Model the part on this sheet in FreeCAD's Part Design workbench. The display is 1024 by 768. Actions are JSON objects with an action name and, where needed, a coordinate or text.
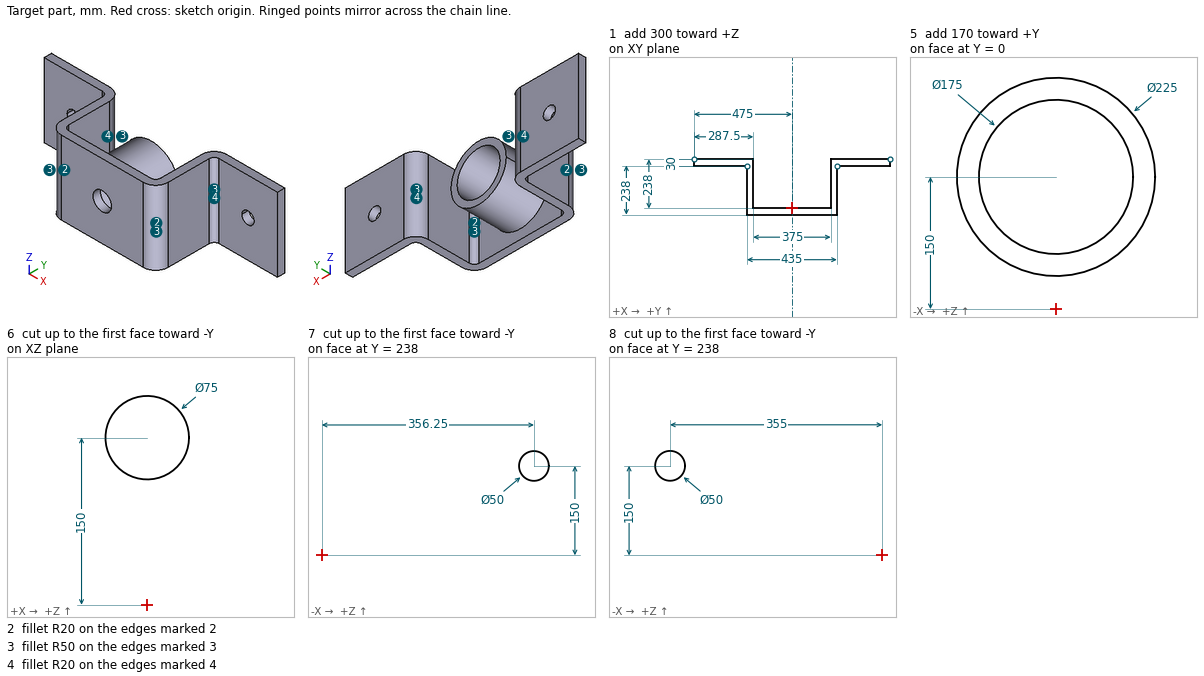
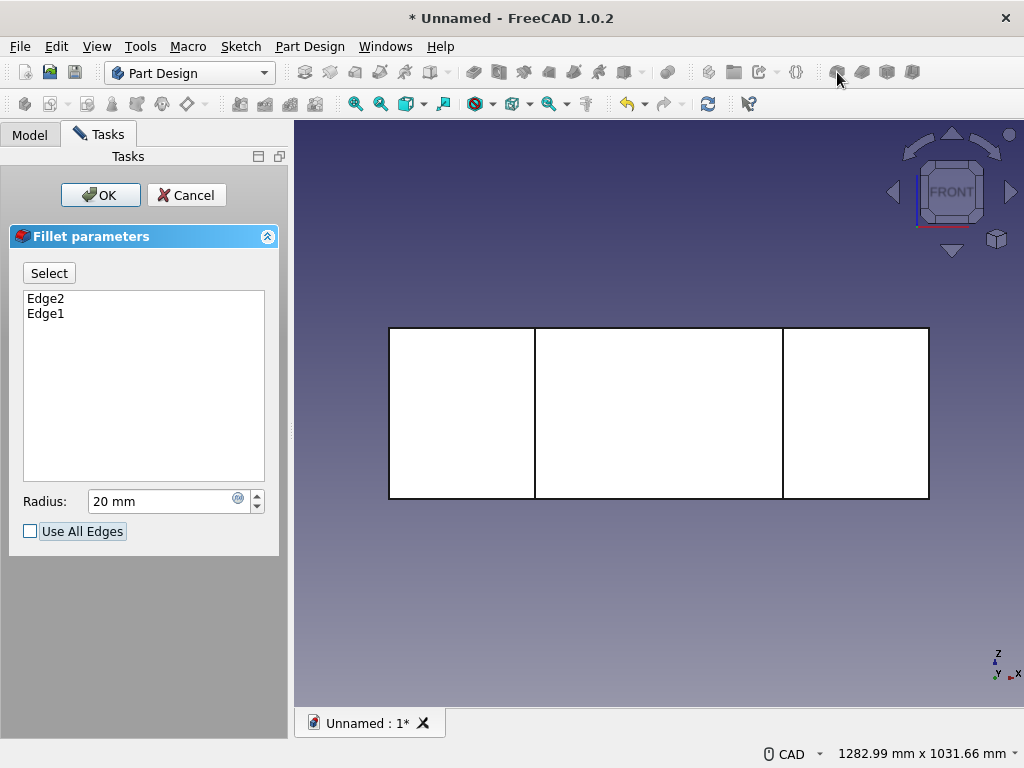
{"action": "left_click", "coordinate": [101, 195]}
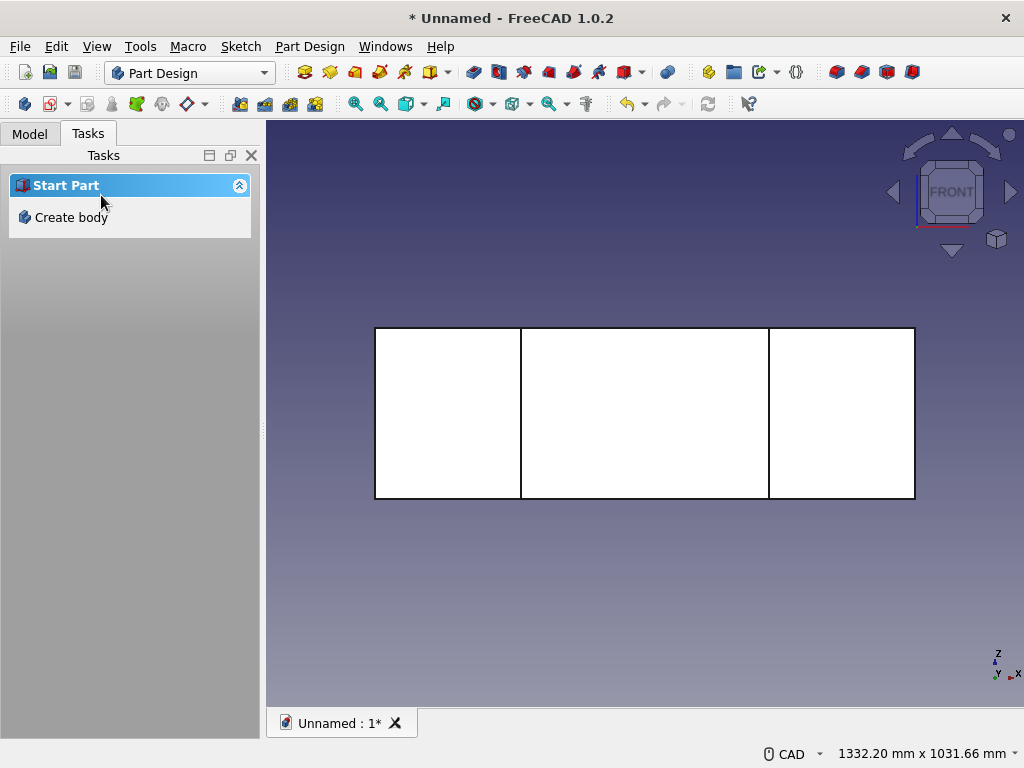
{"action": "left_click", "coordinate": [769, 412]}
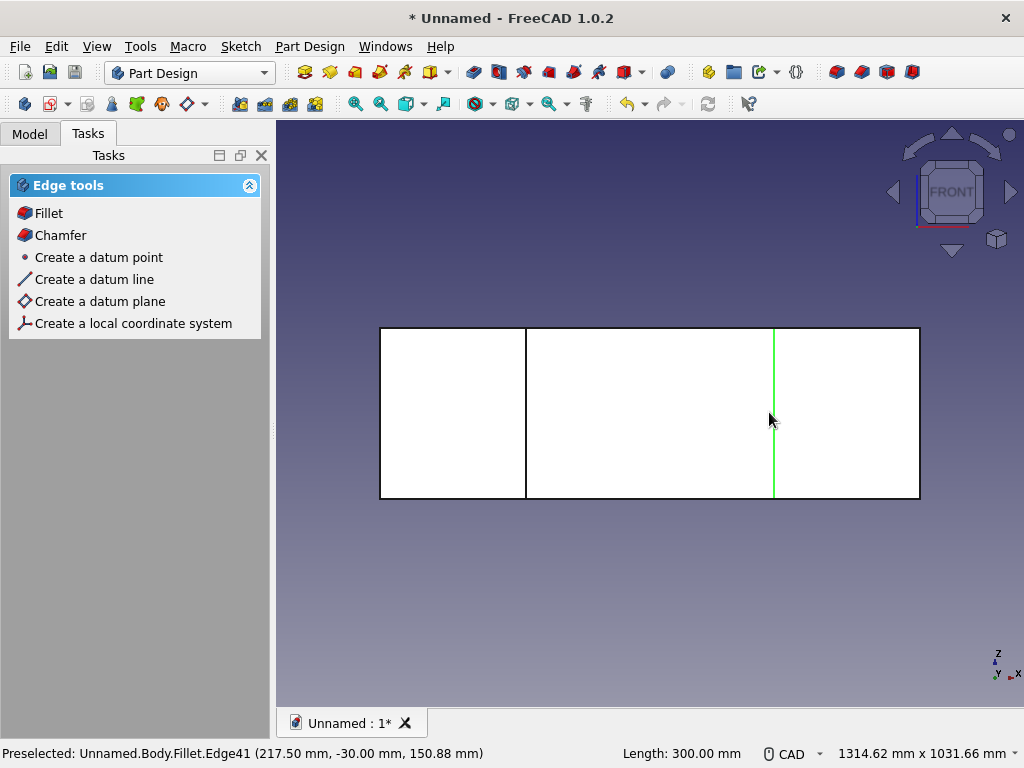
{"action": "left_click", "coordinate": [526, 412], "text": "ctrl"}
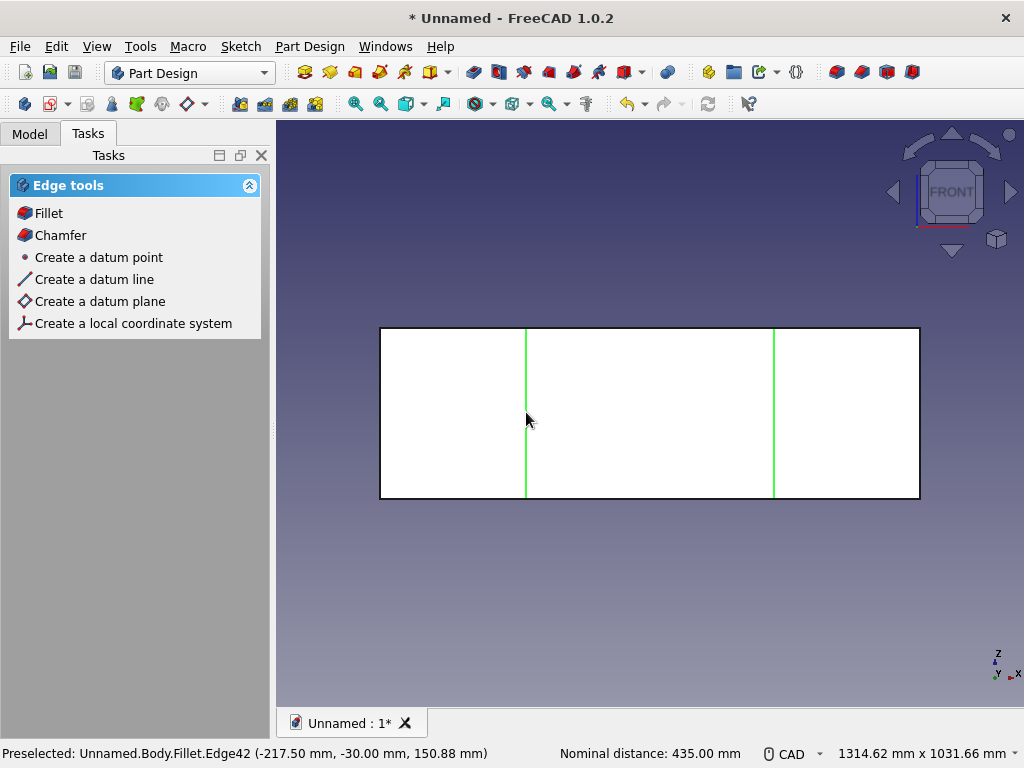
{"action": "key", "text": "0"}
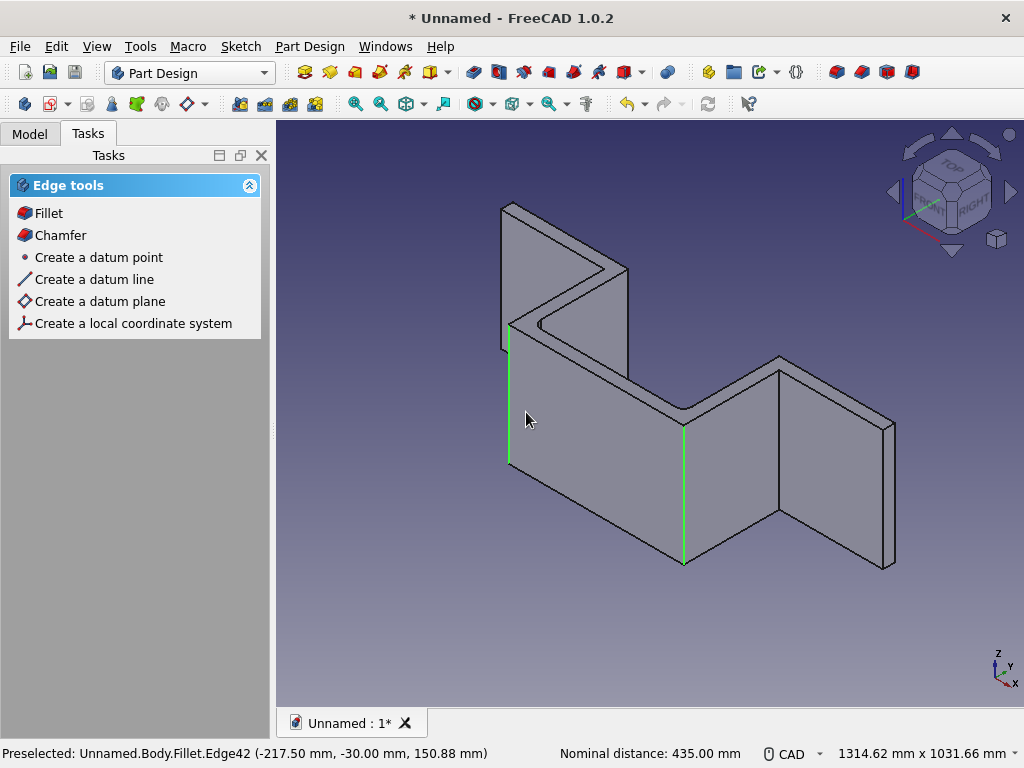
{"action": "key", "text": "2"}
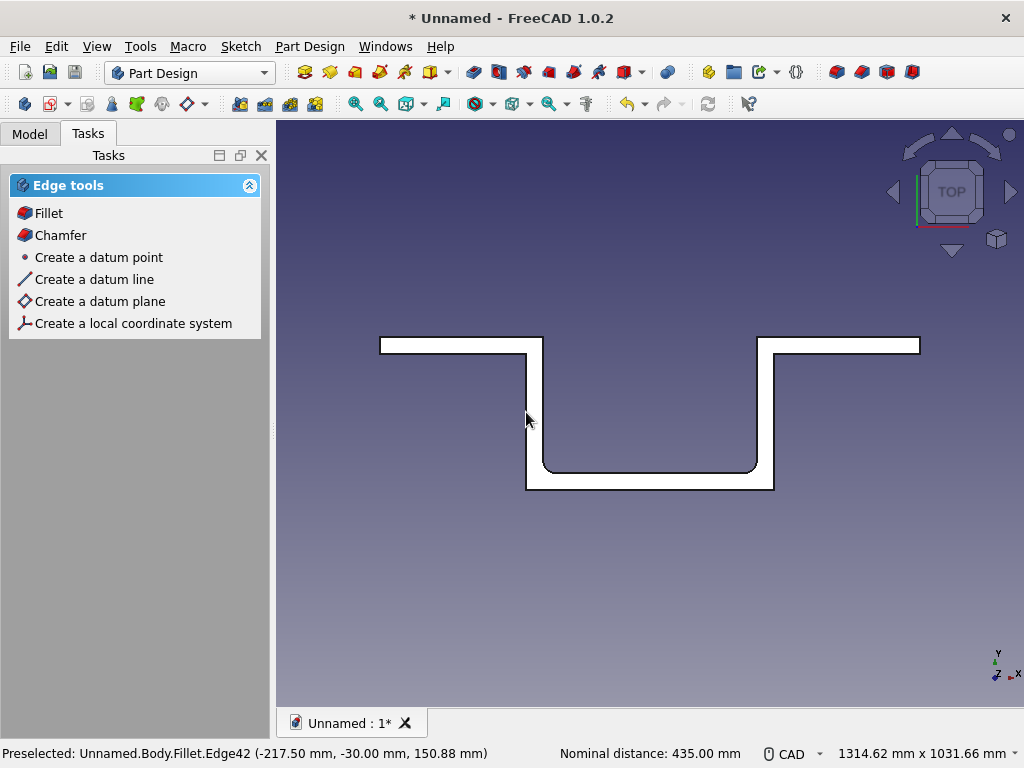
{"action": "key", "text": "1"}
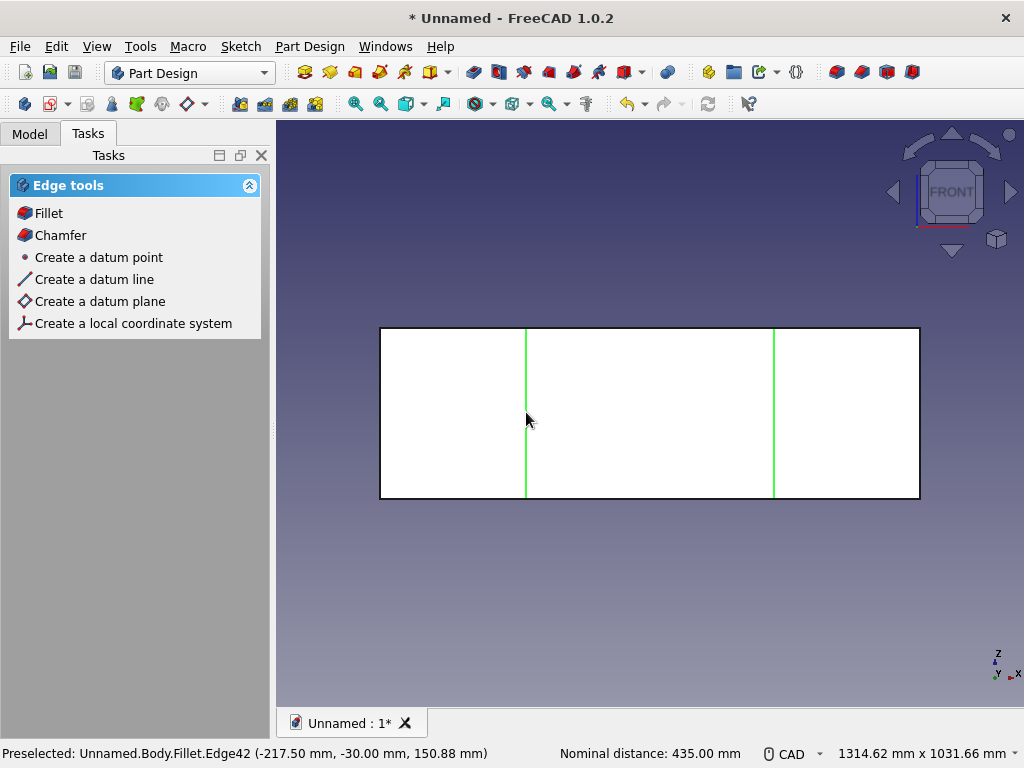
{"action": "key", "text": "3"}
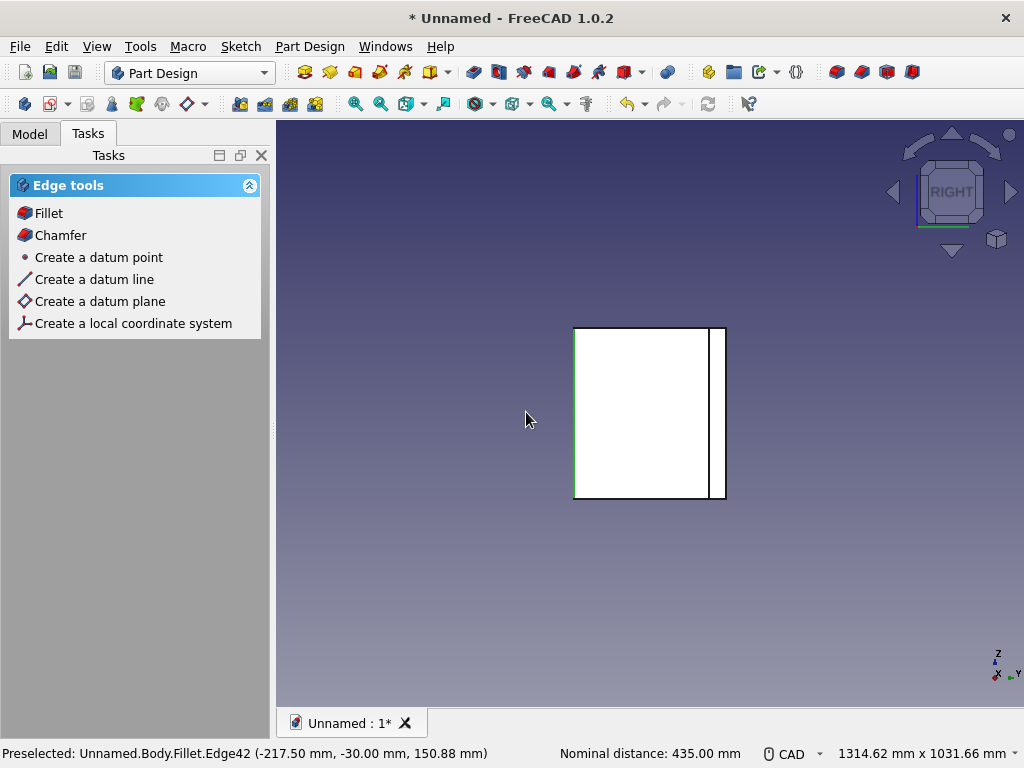
{"action": "left_click", "coordinate": [356, 104]}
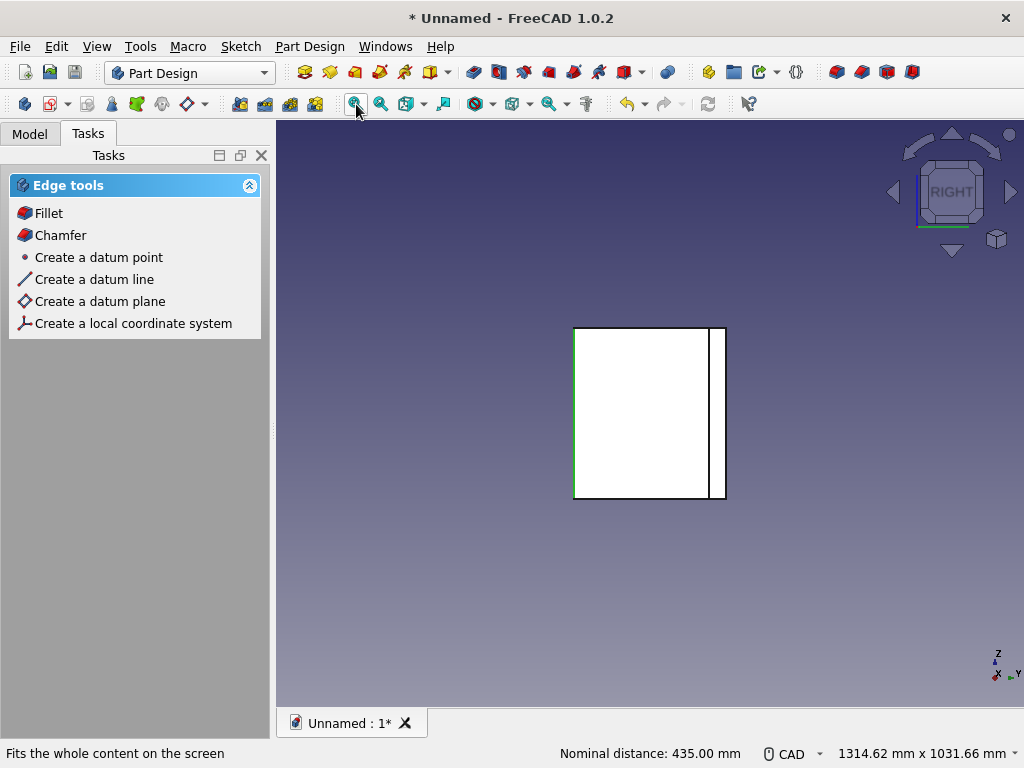
{"action": "key", "text": "5"}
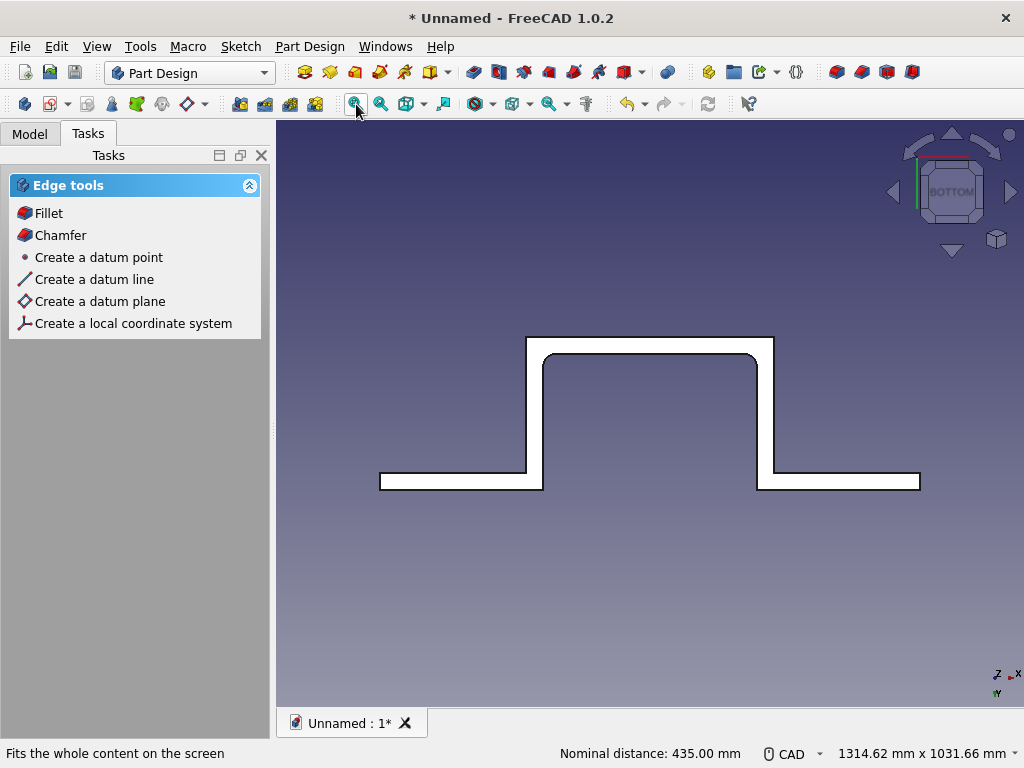
{"action": "key", "text": "4"}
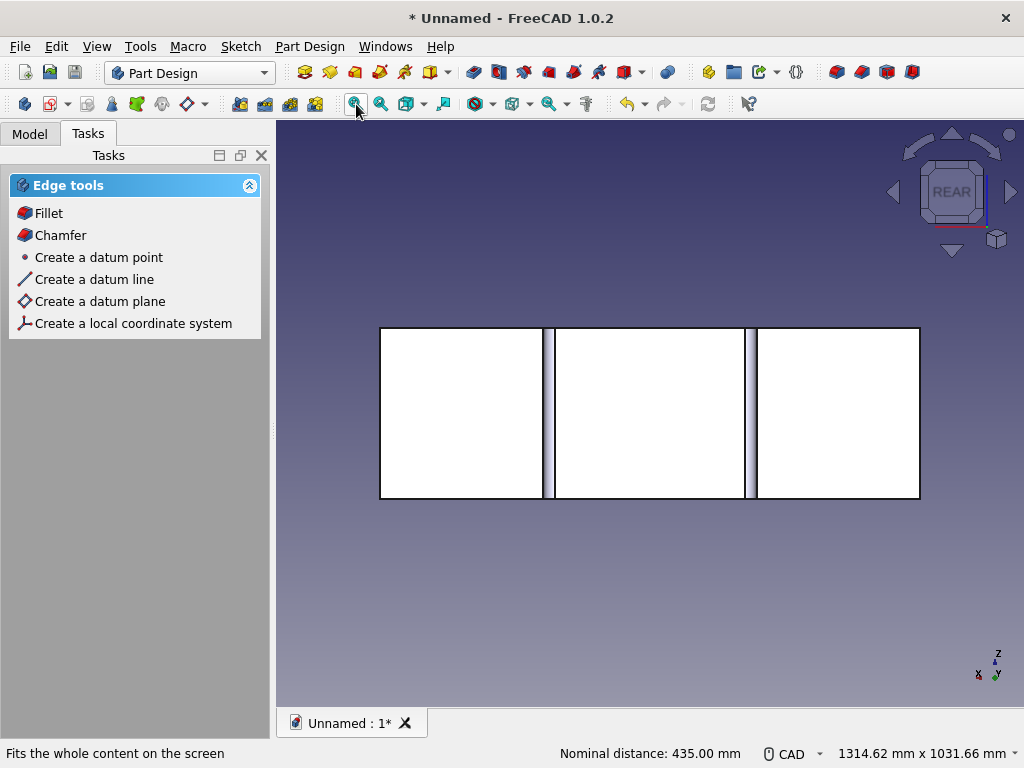
{"action": "left_click", "coordinate": [543, 412], "text": "ctrl"}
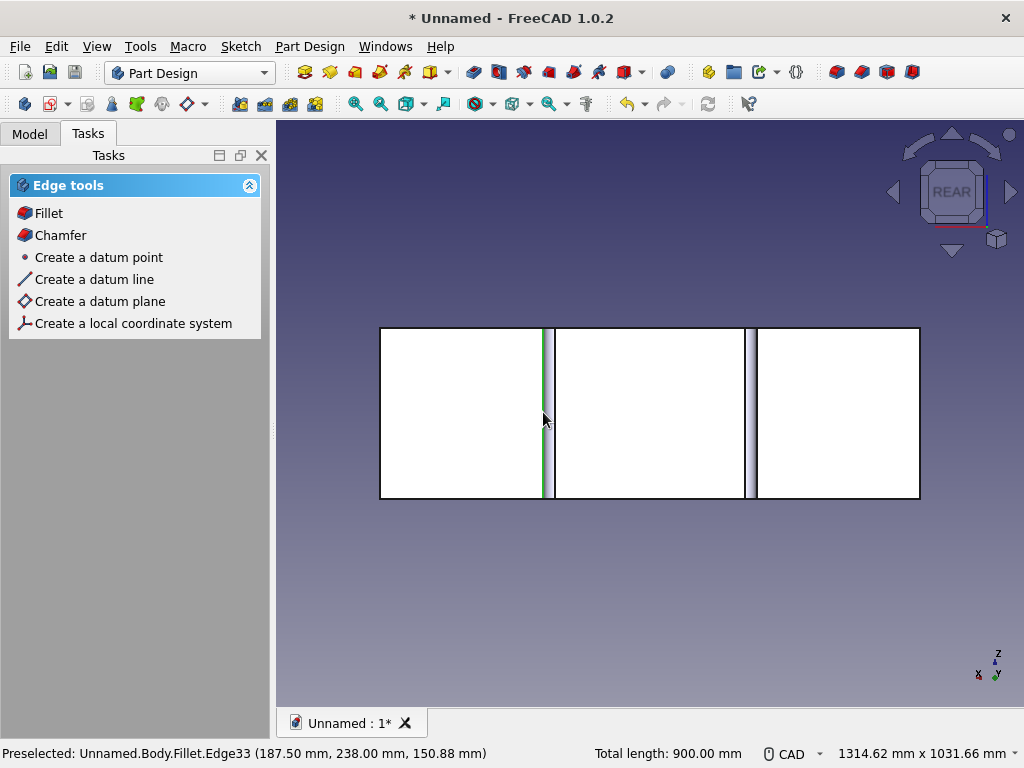
{"action": "left_click", "coordinate": [757, 412], "text": "ctrl"}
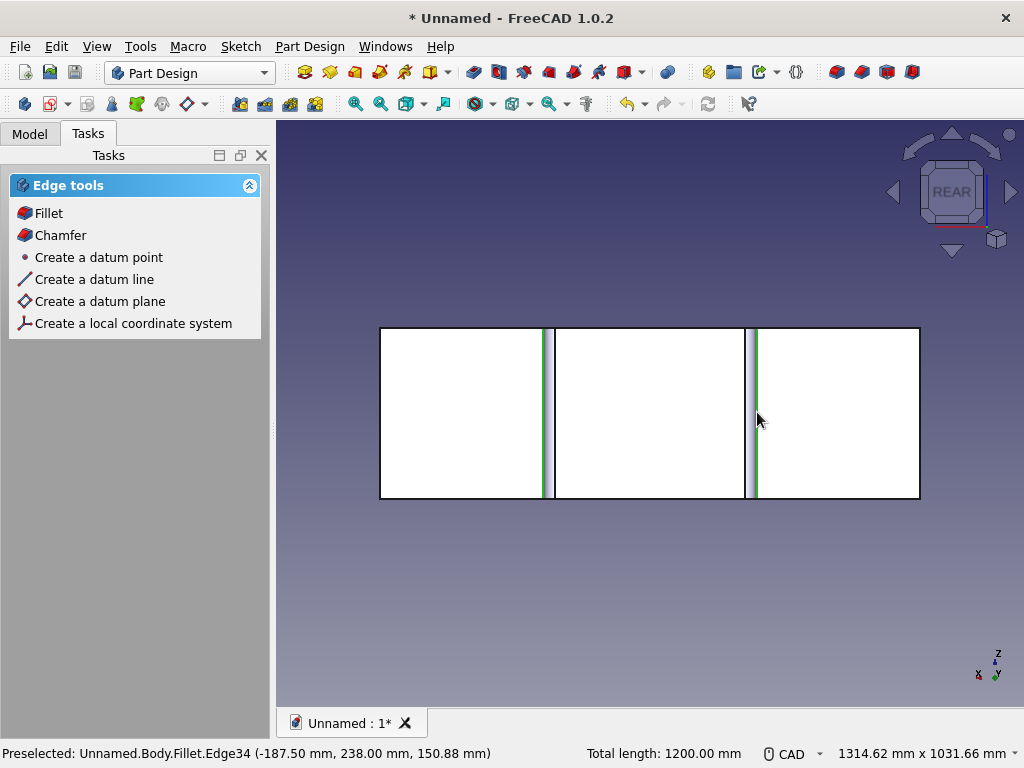
{"action": "left_click", "coordinate": [837, 72]}